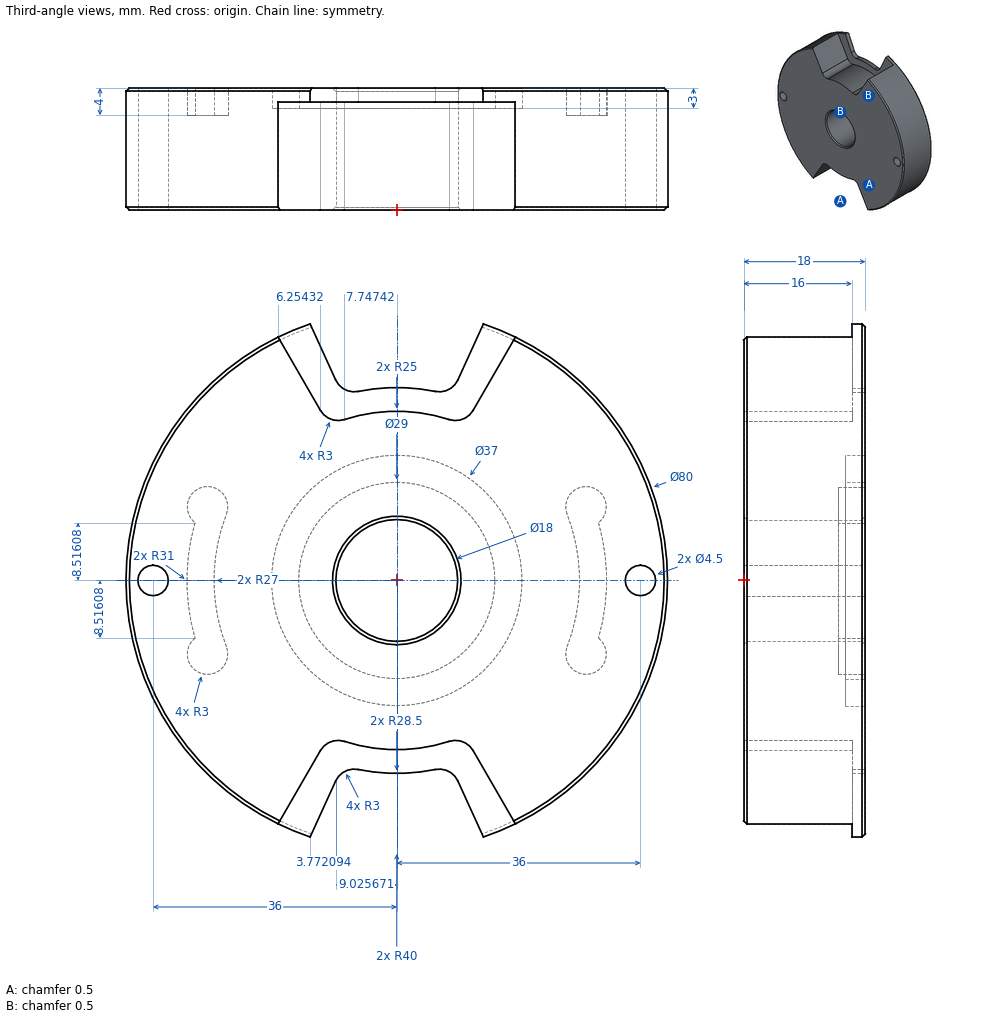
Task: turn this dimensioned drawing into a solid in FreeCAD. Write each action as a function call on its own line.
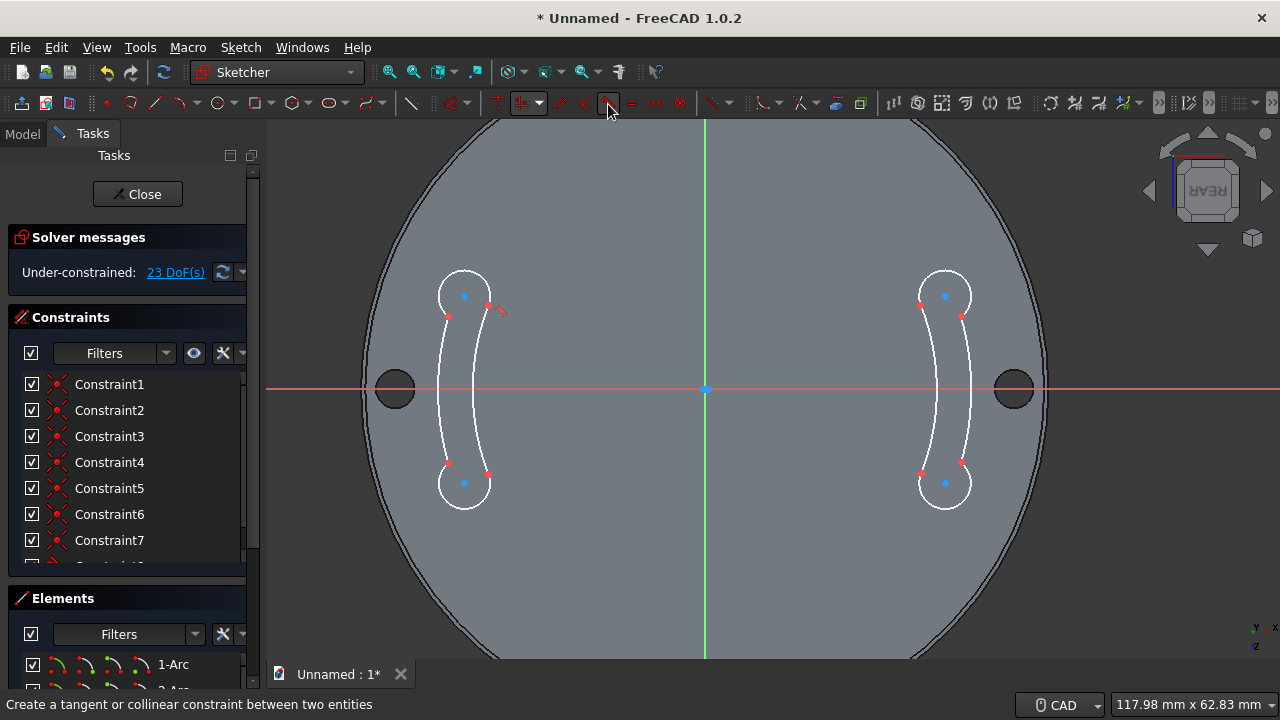
click(475, 356)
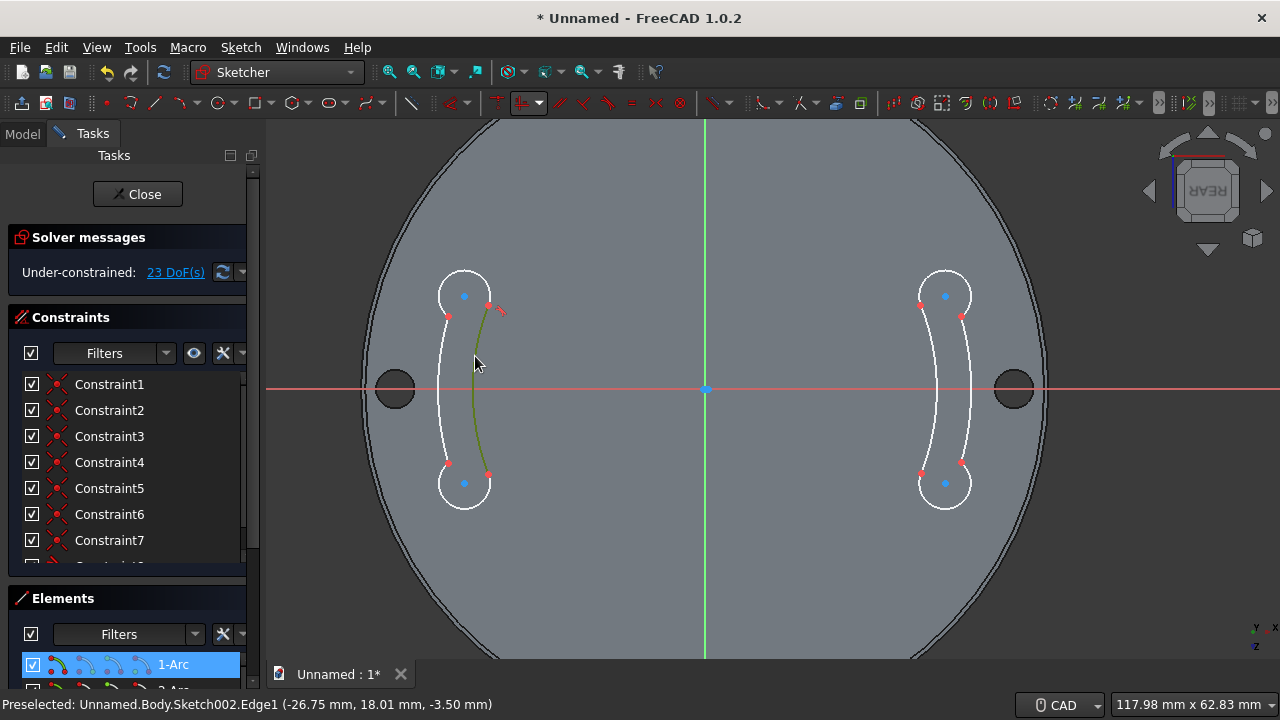
click(441, 494)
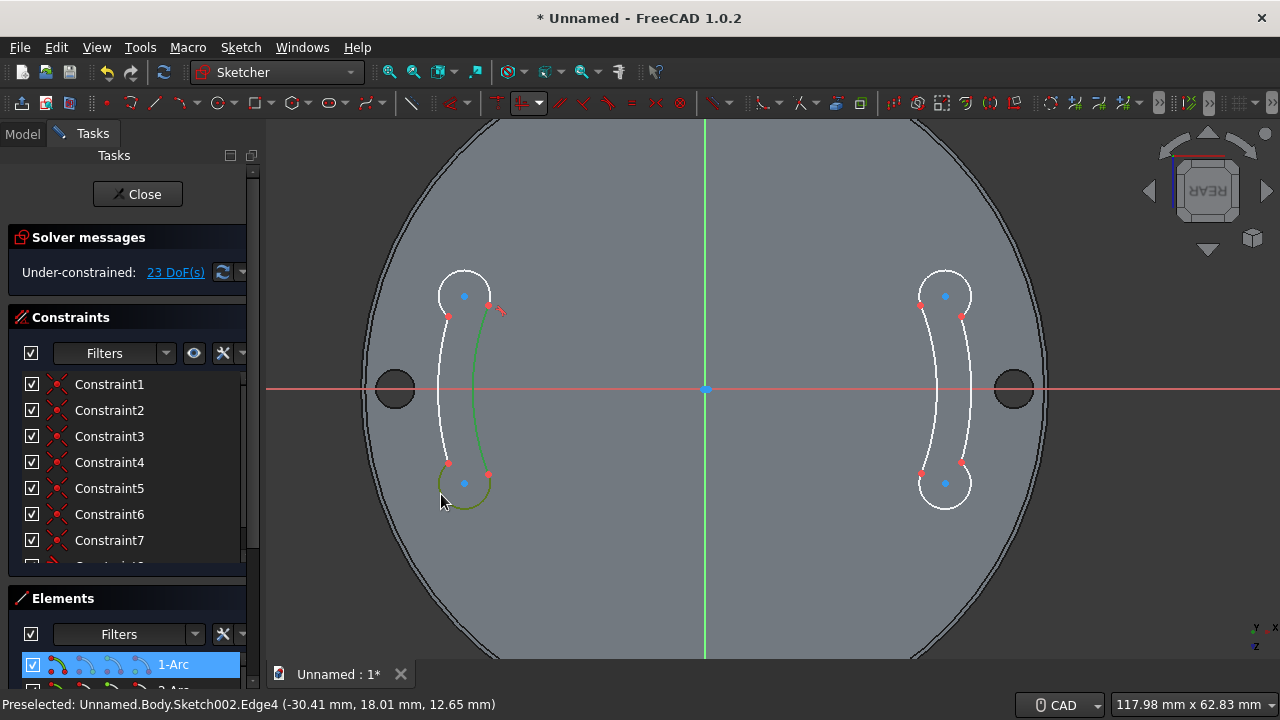
click(608, 104)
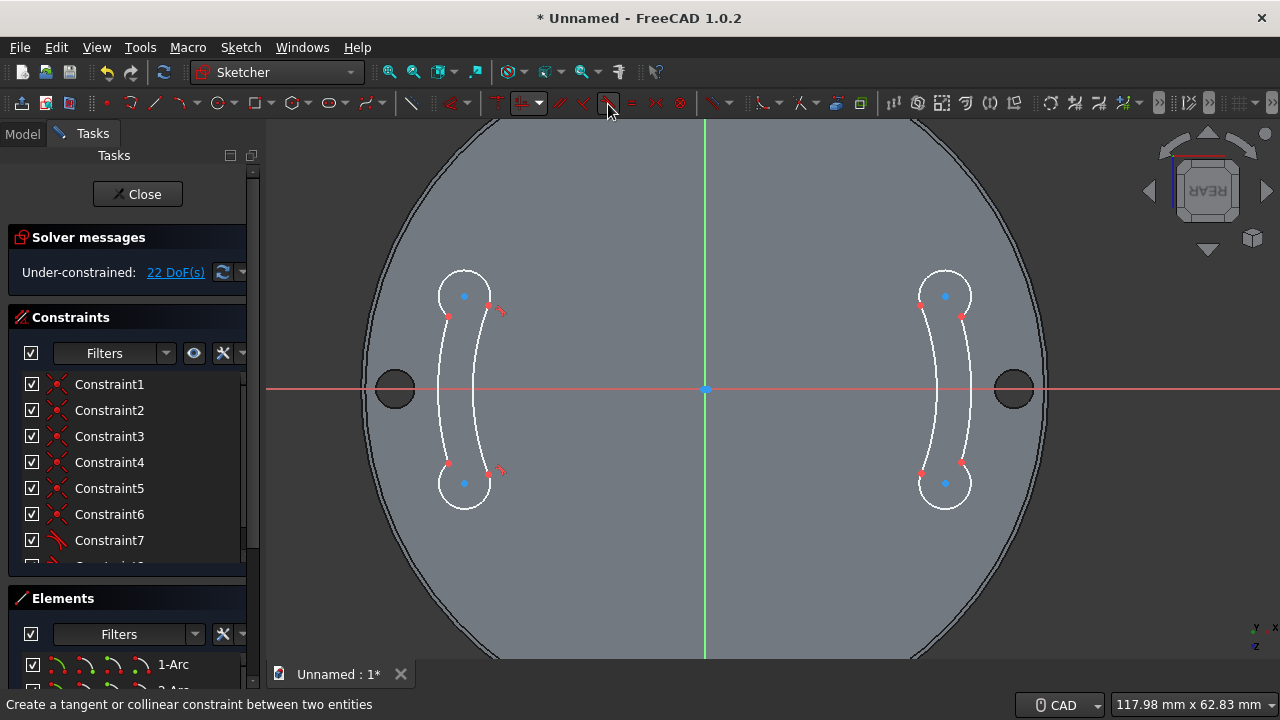
click(930, 504)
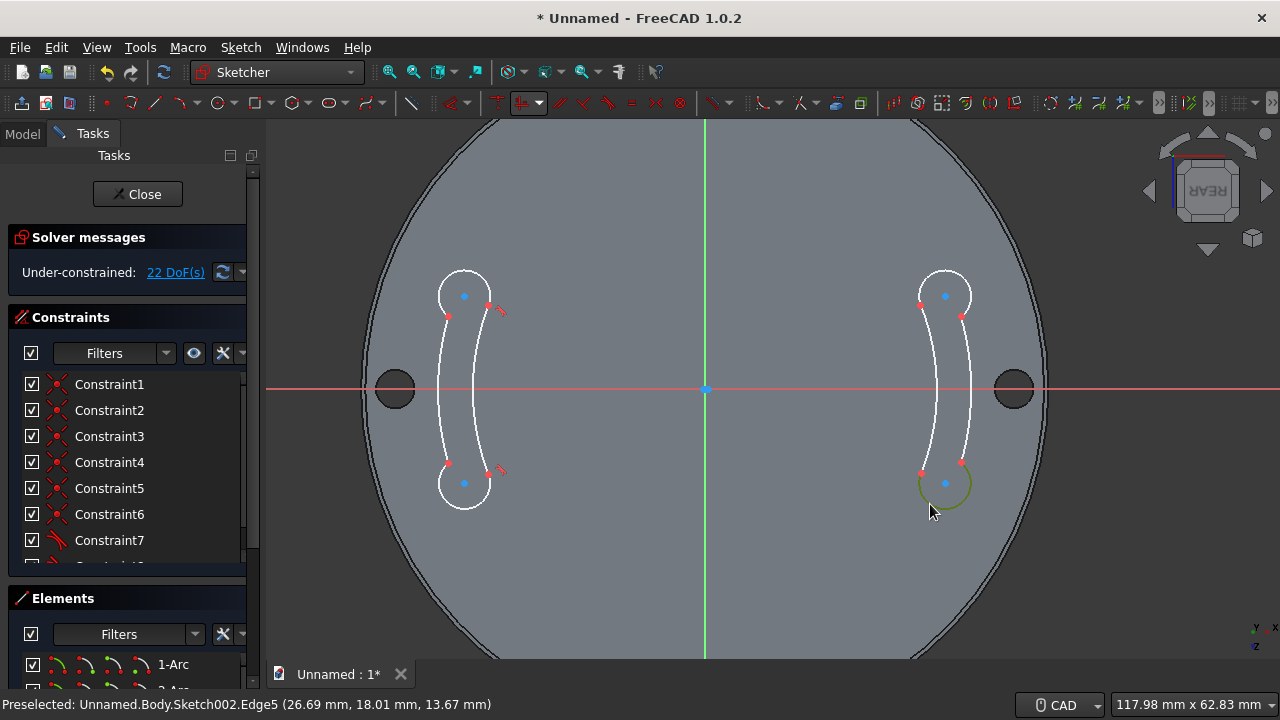
click(934, 424)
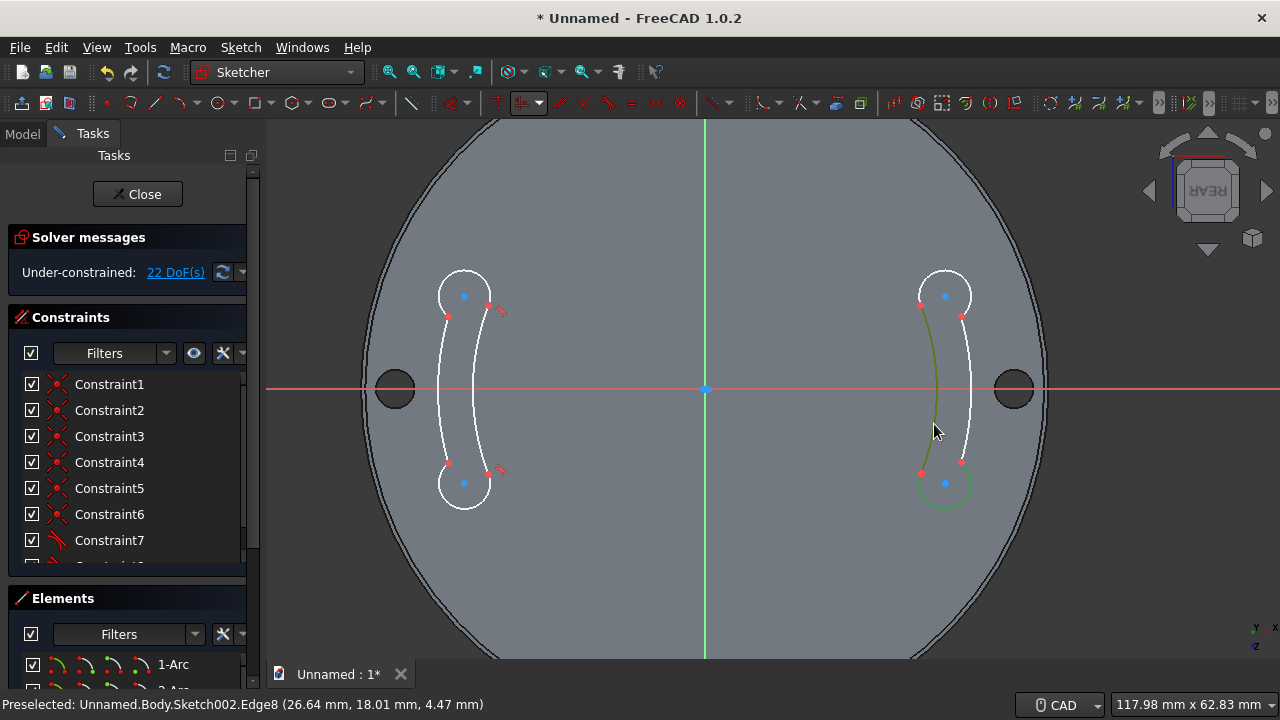
click(608, 104)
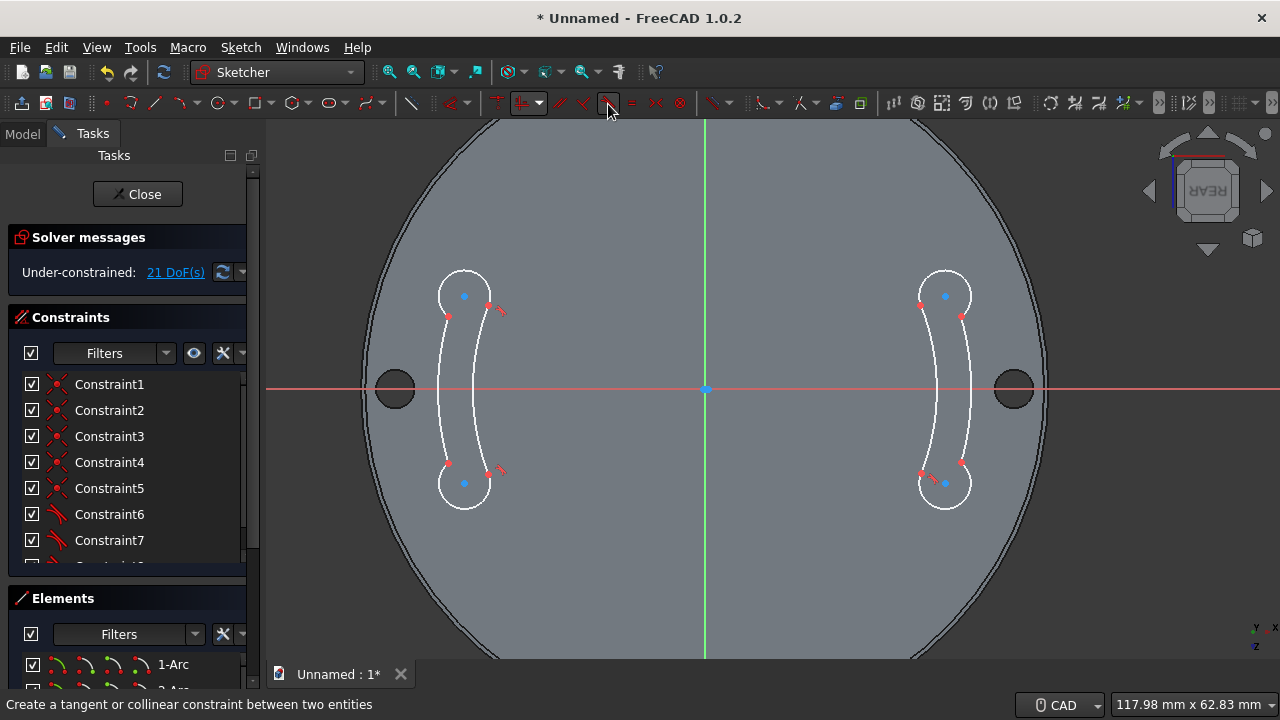
click(969, 286)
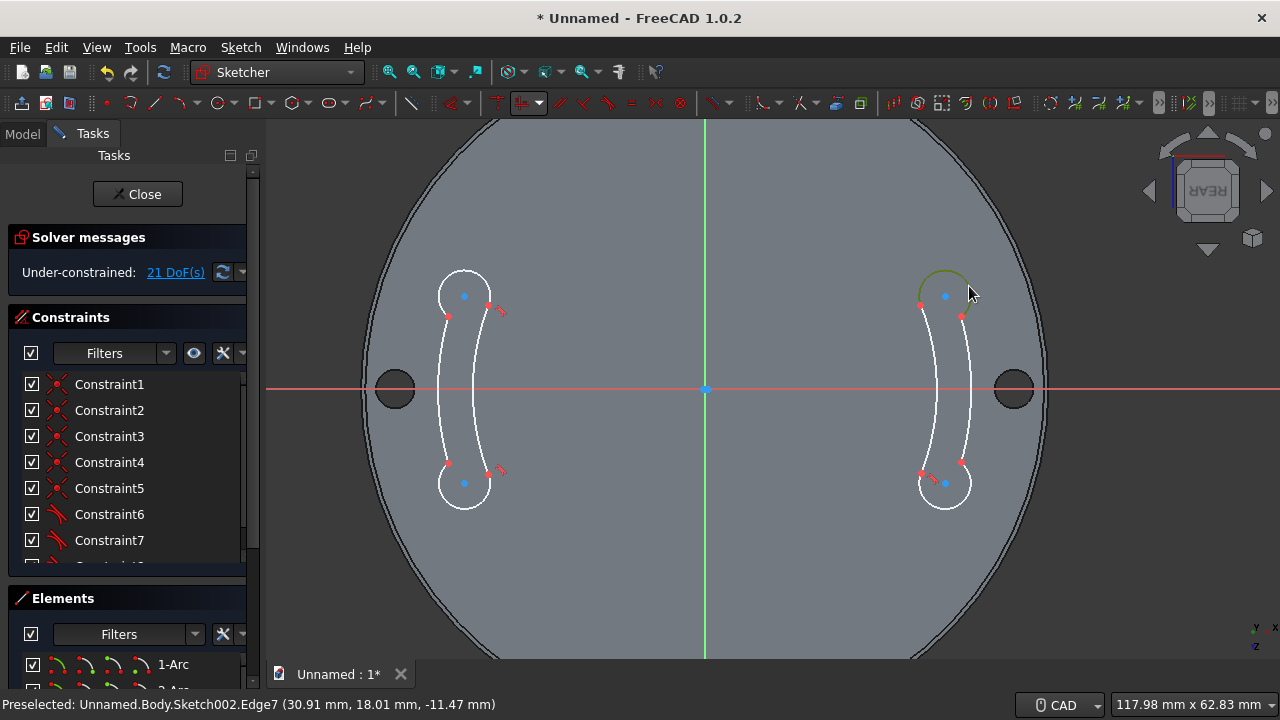
click(934, 424)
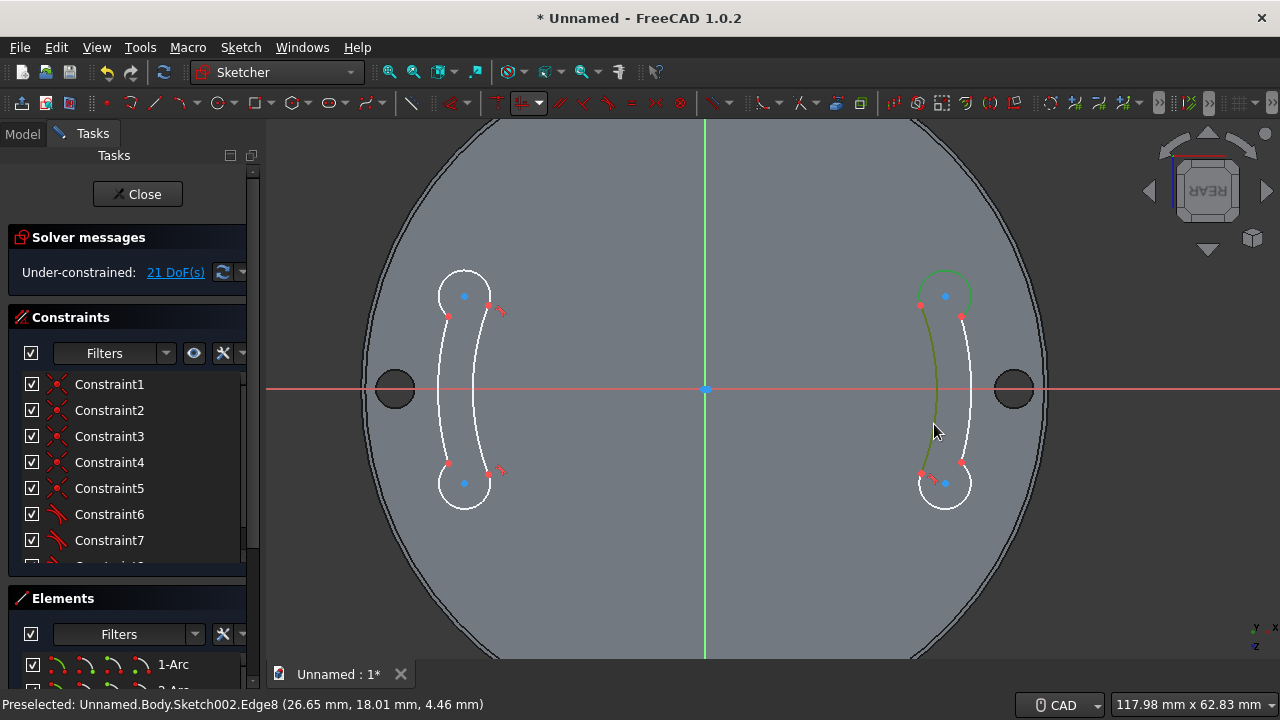
click(608, 104)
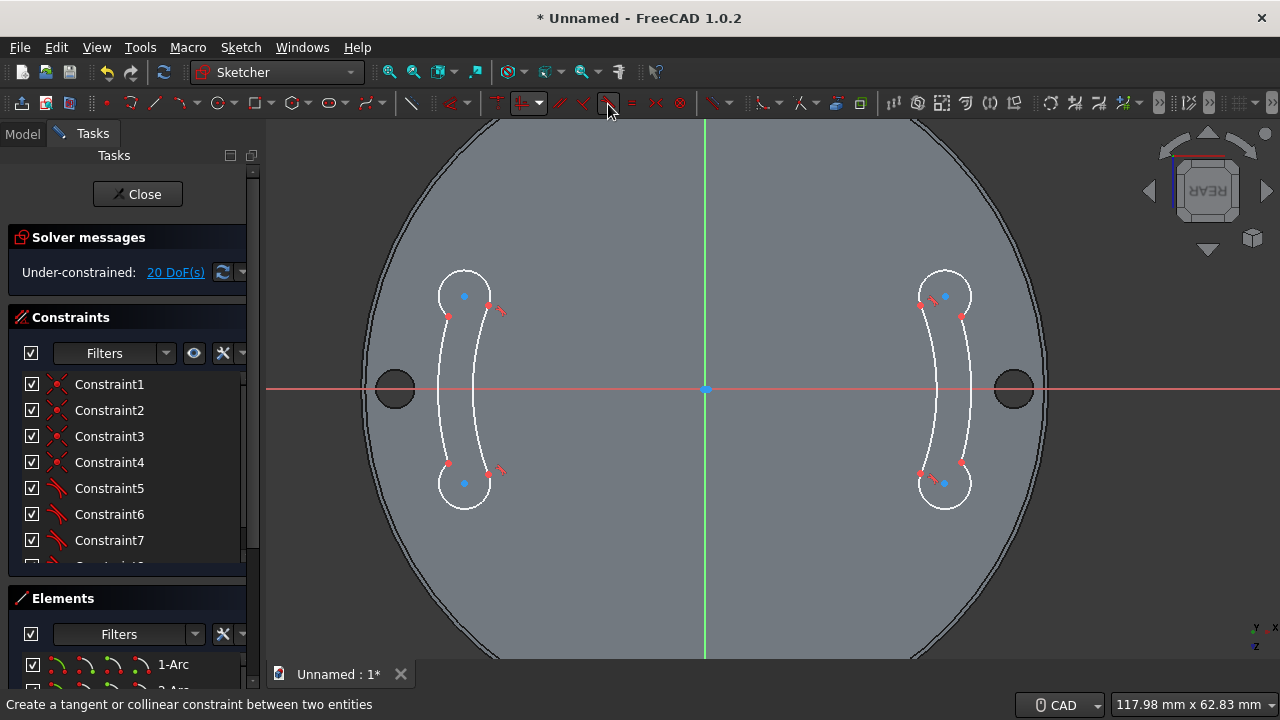
click(475, 355)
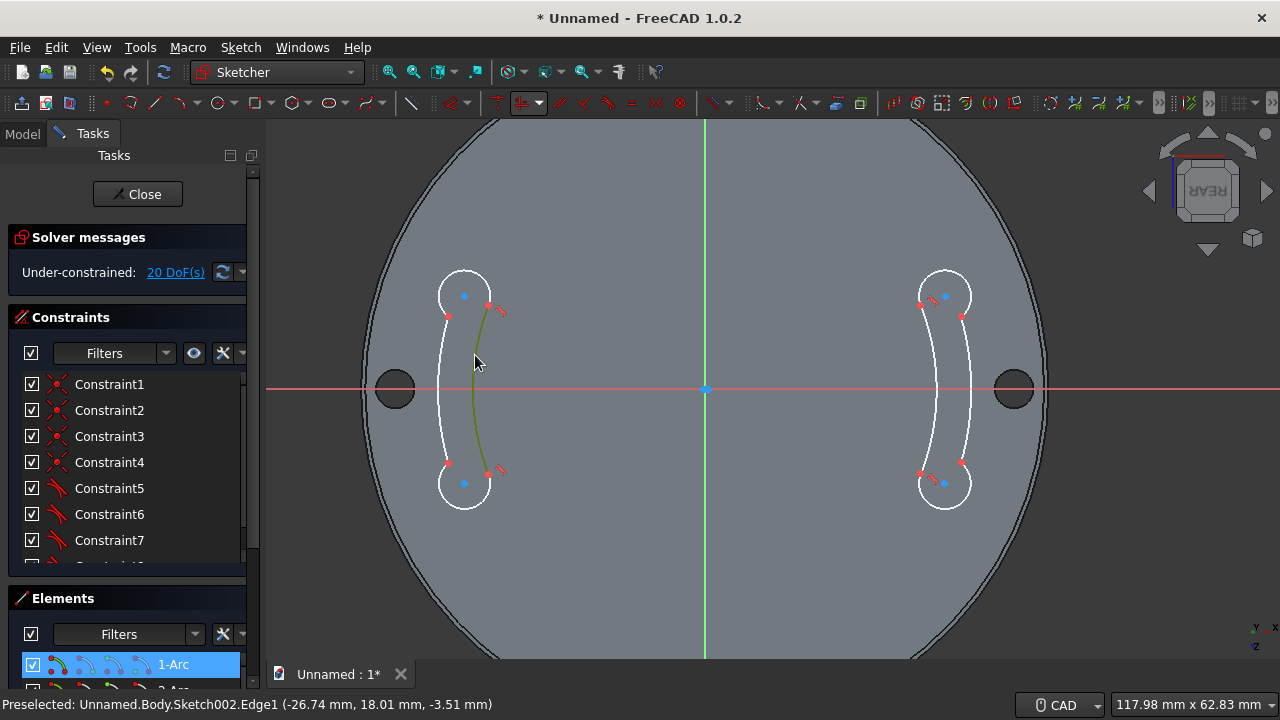
click(440, 360)